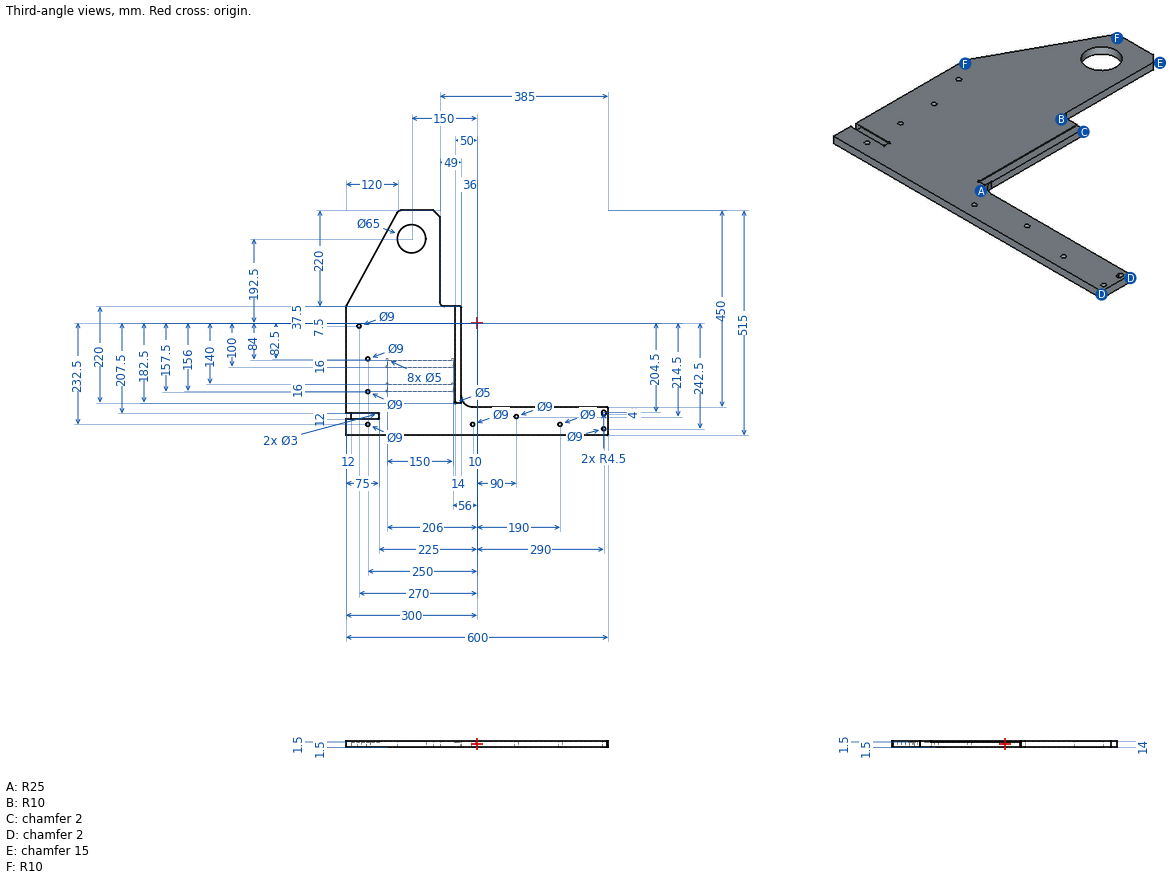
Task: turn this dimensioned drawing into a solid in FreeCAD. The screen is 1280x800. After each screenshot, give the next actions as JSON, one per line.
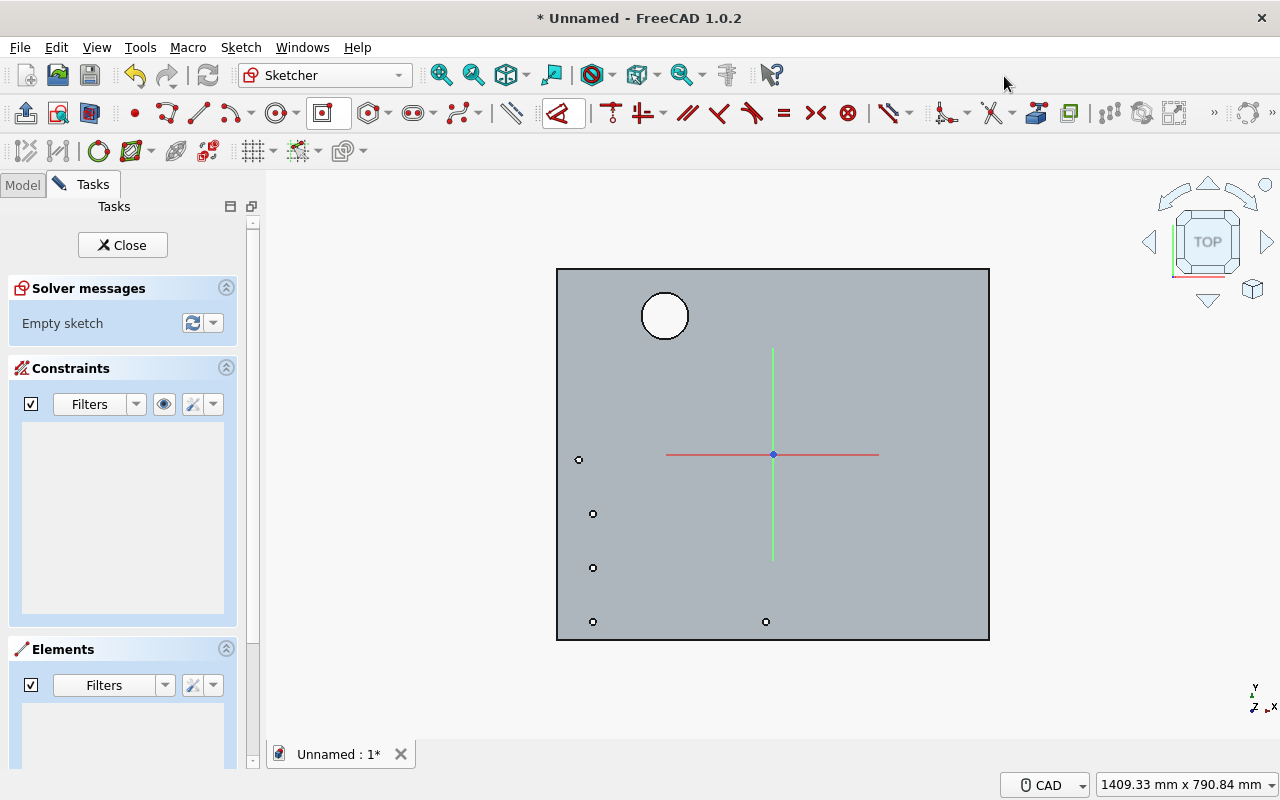
{"action": "scroll", "coordinate": [572, 623], "scroll_direction": "up", "scroll_amount": 12}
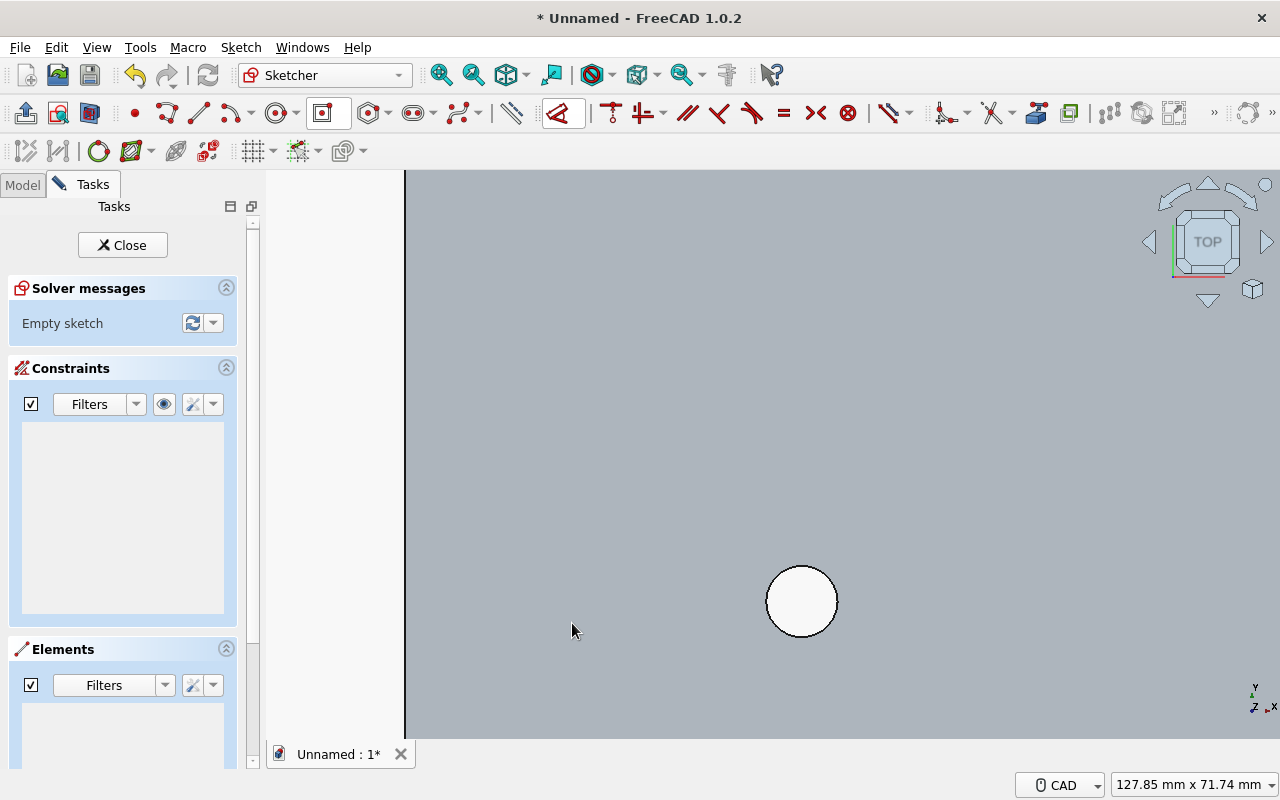
{"action": "key", "text": "g r"}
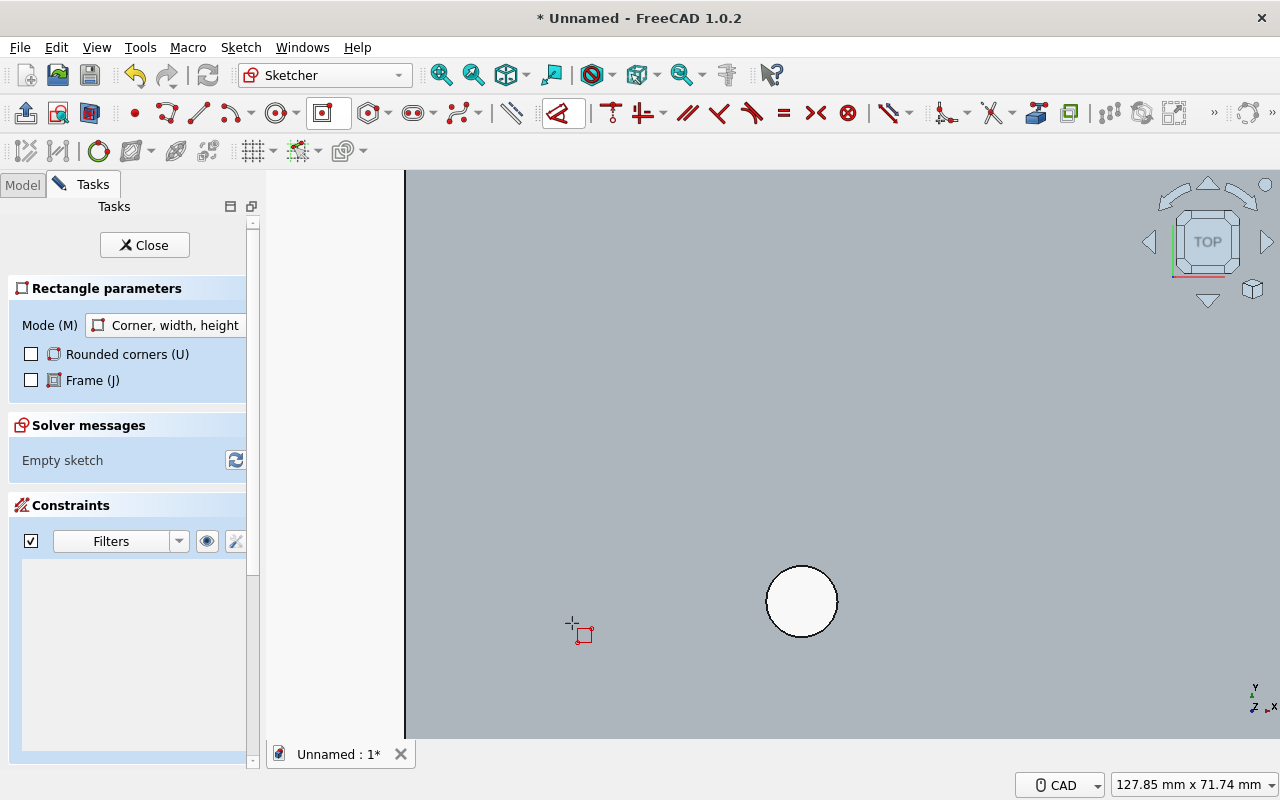
{"action": "left_click", "coordinate": [405, 403]}
{"action": "mouse_move", "coordinate": [1000, 498]}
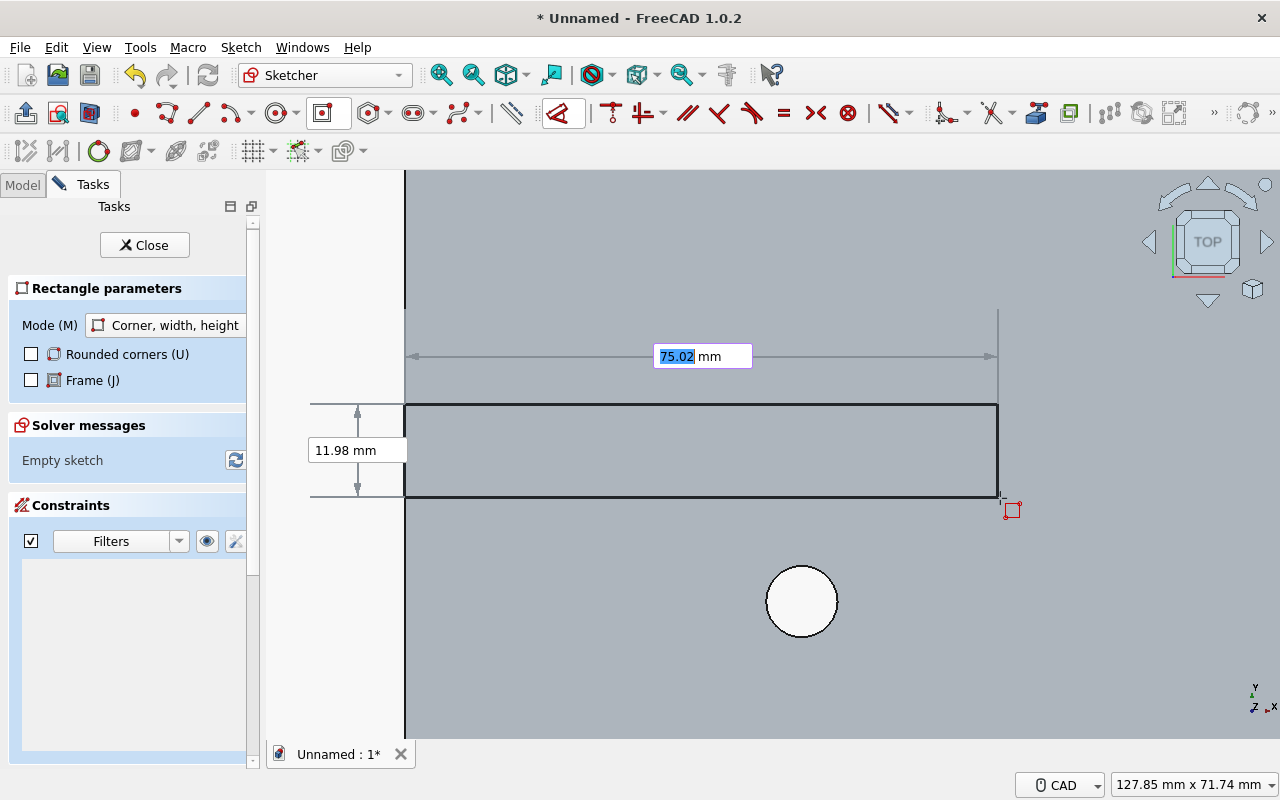
{"action": "type", "text": "75"}
{"action": "key", "text": "Tab"}
{"action": "type", "text": "12"}
{"action": "key", "text": "Return"}
{"action": "key", "text": "Escape"}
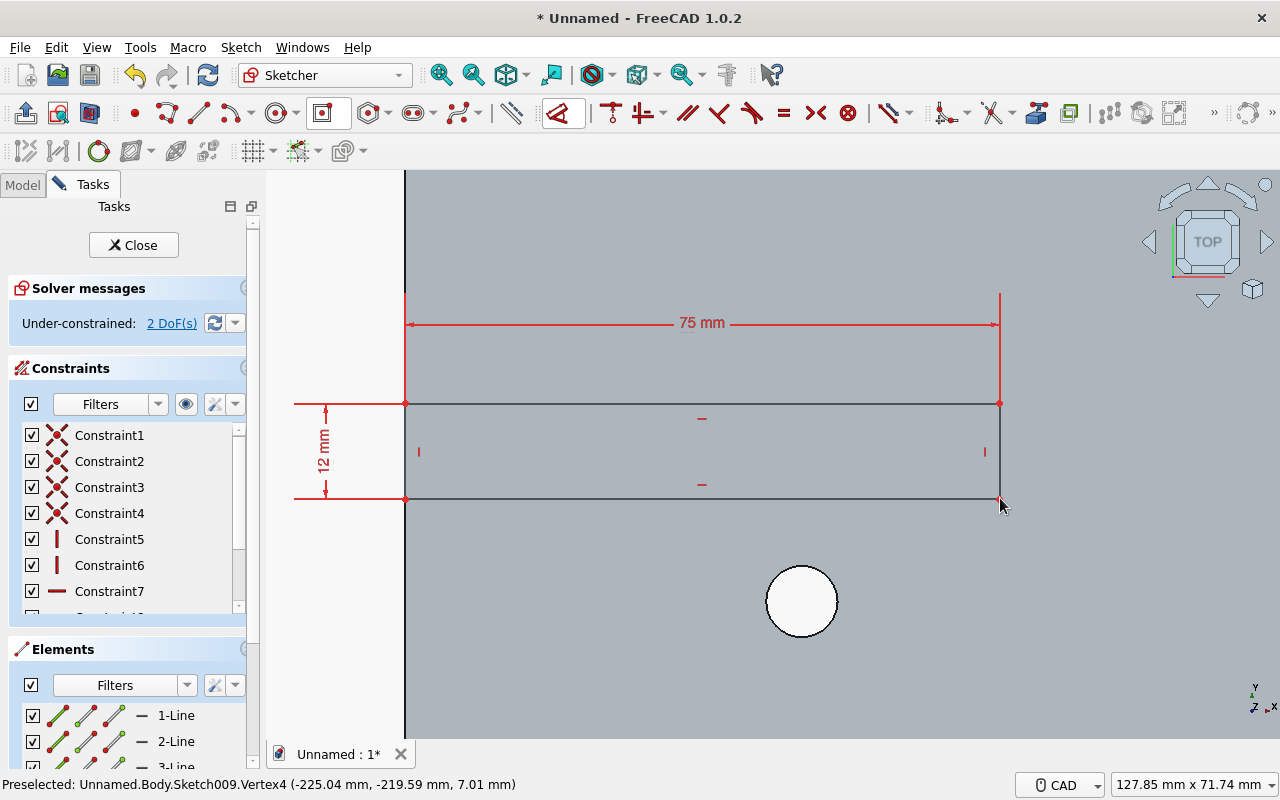
{"action": "left_click", "coordinate": [405, 404]}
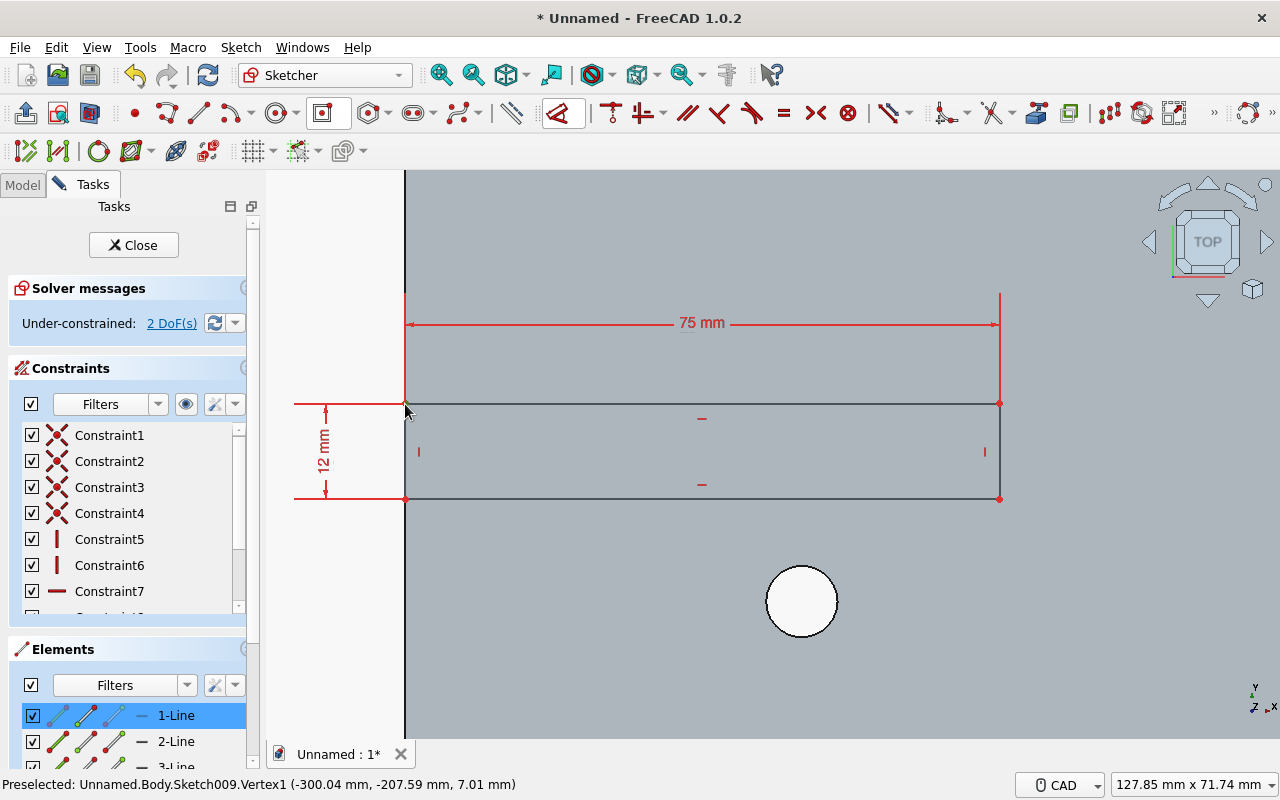
{"action": "key", "text": "l"}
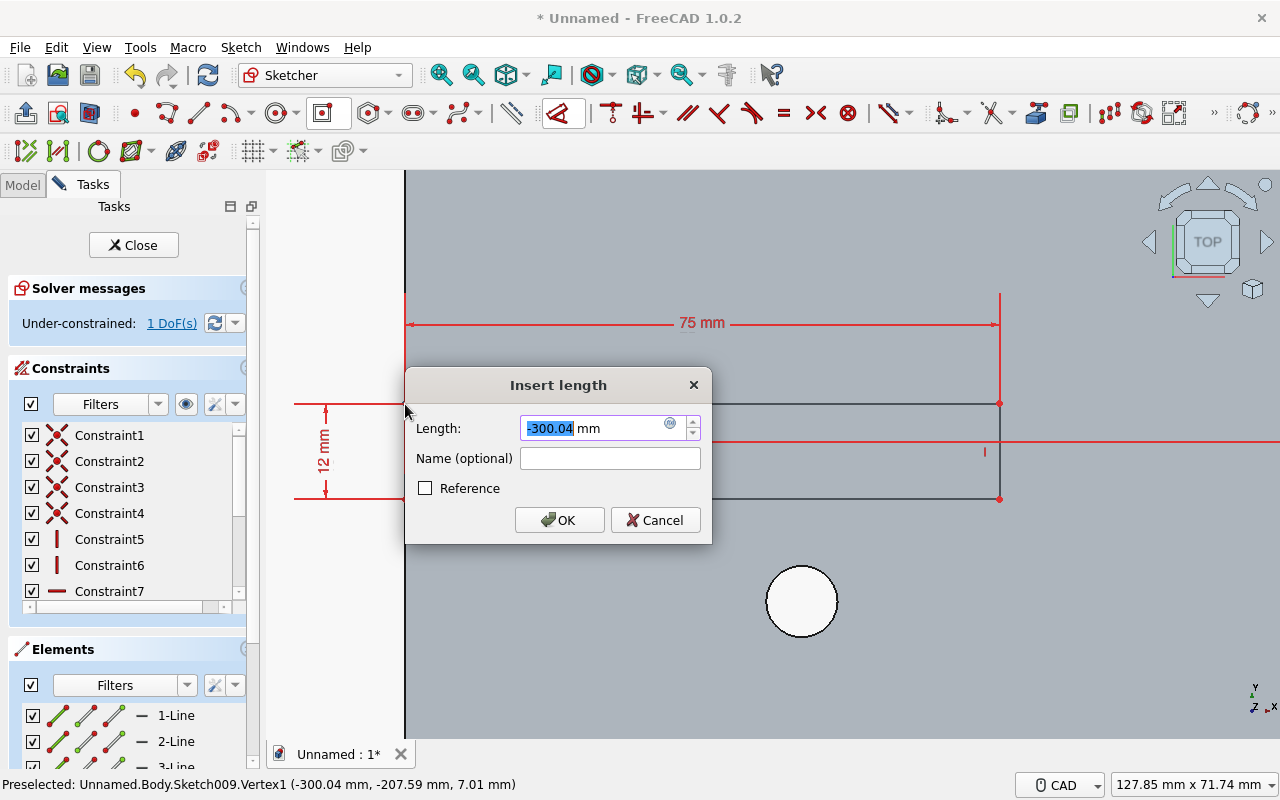
{"action": "type", "text": "-300"}
{"action": "key", "text": "Return"}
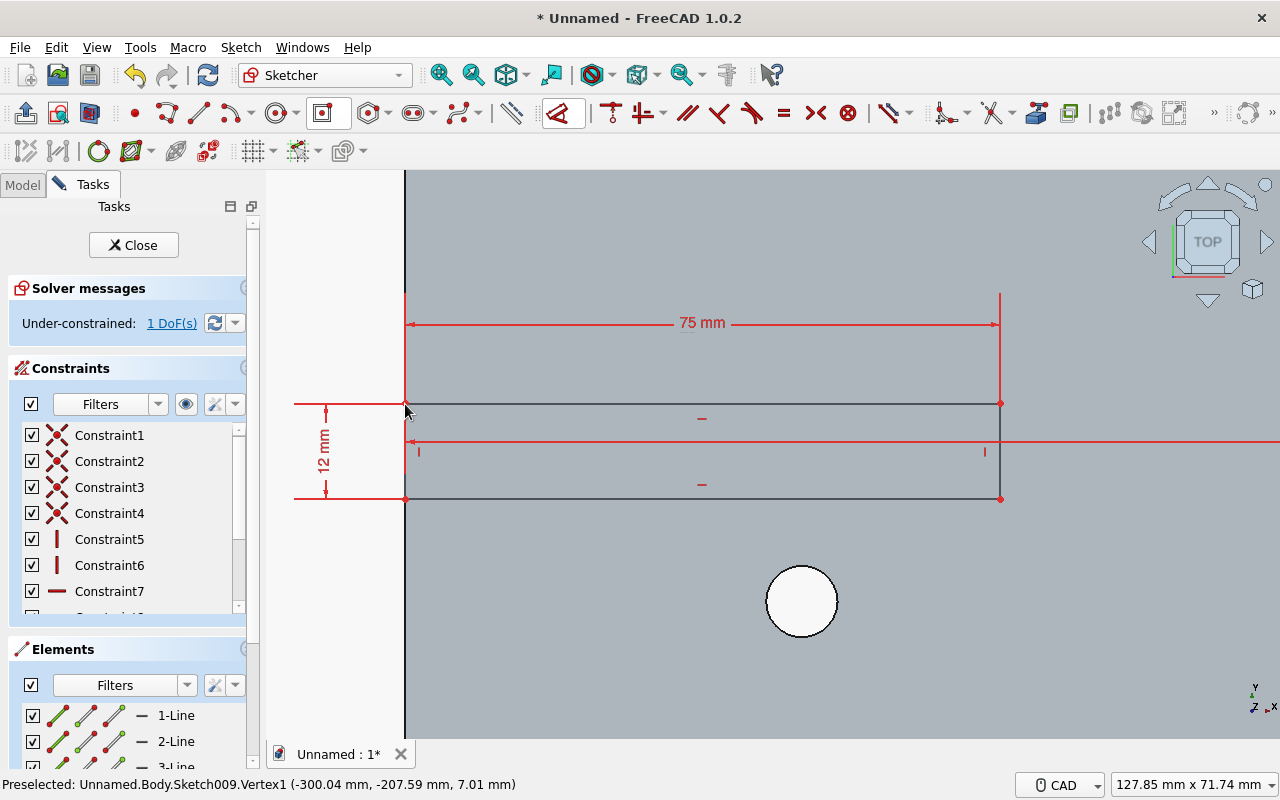
{"action": "left_click", "coordinate": [405, 404]}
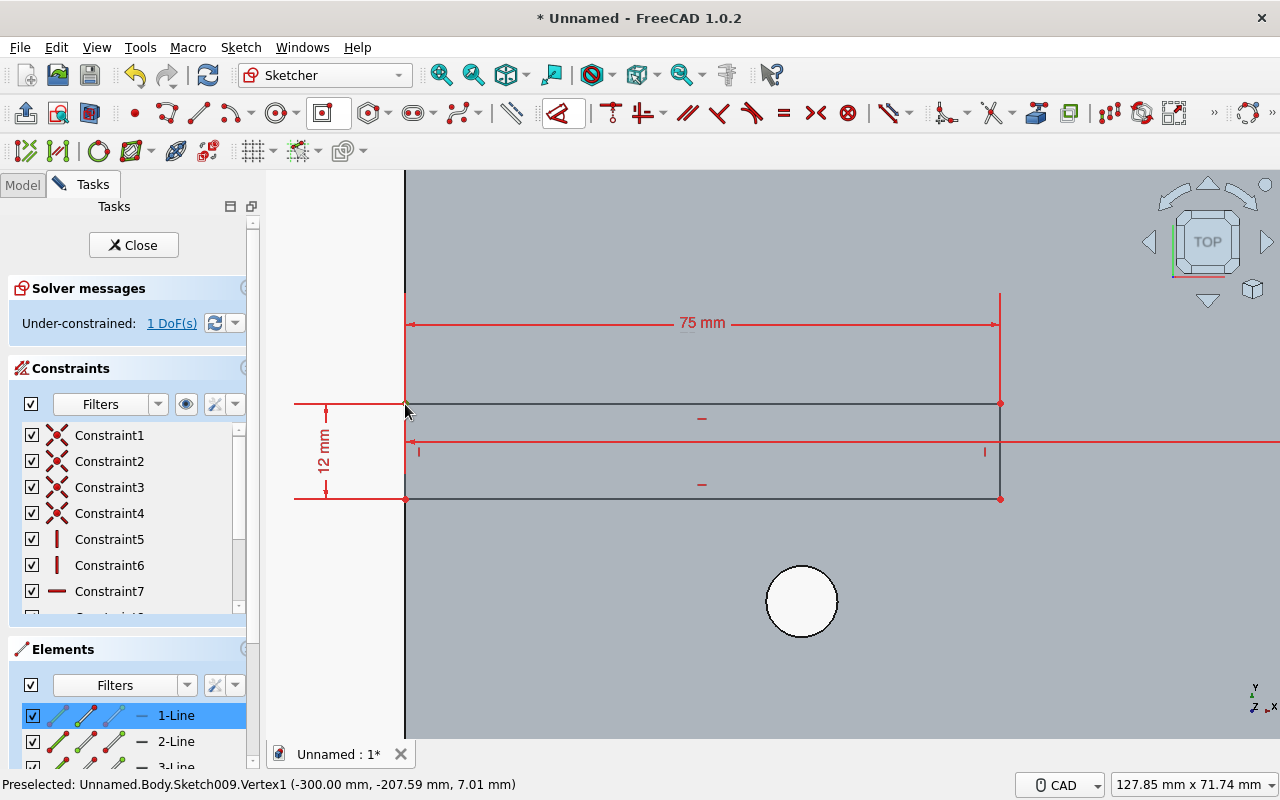
{"action": "left_click", "coordinate": [580, 114]}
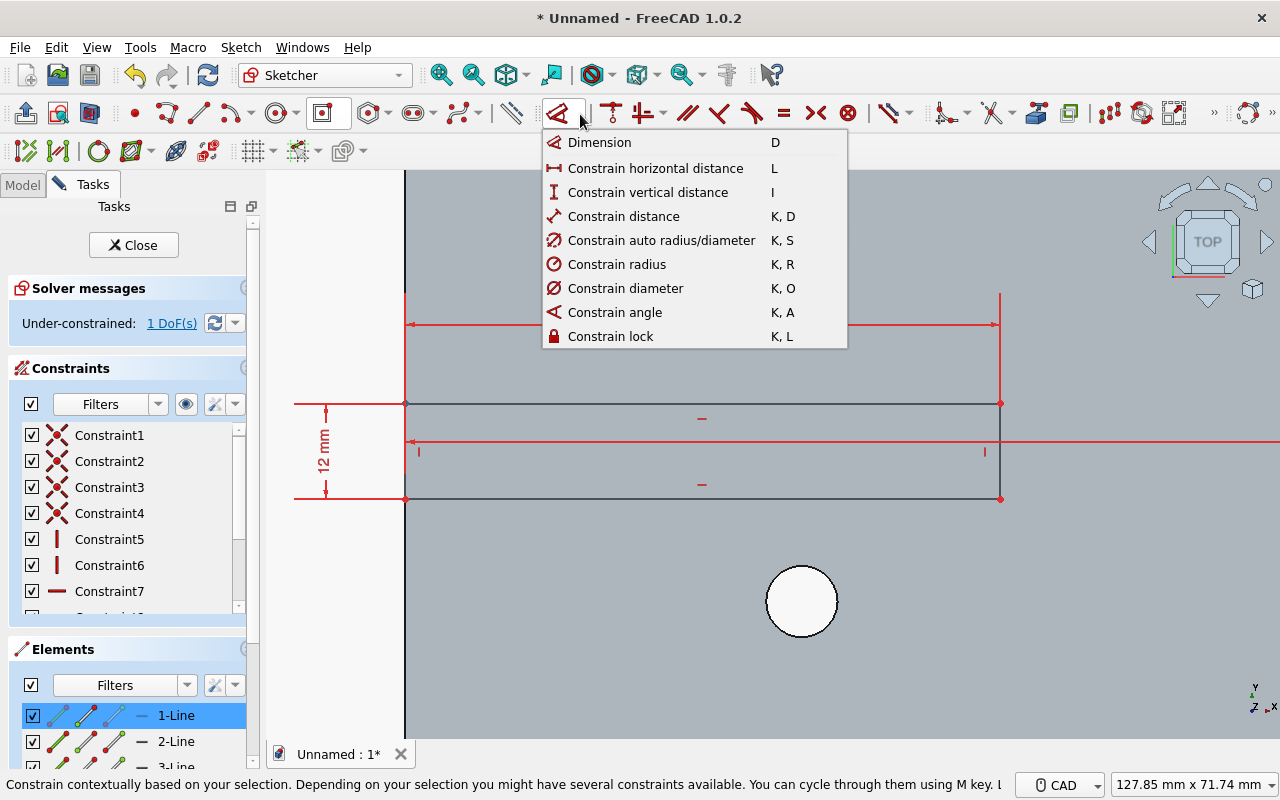
{"action": "left_click", "coordinate": [695, 192]}